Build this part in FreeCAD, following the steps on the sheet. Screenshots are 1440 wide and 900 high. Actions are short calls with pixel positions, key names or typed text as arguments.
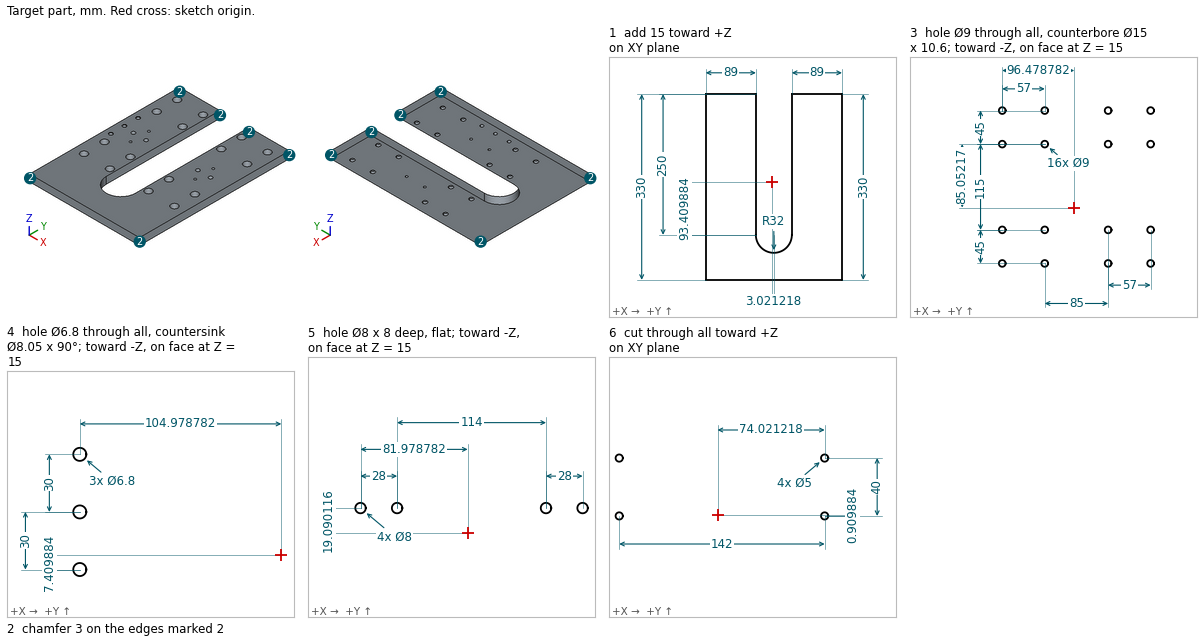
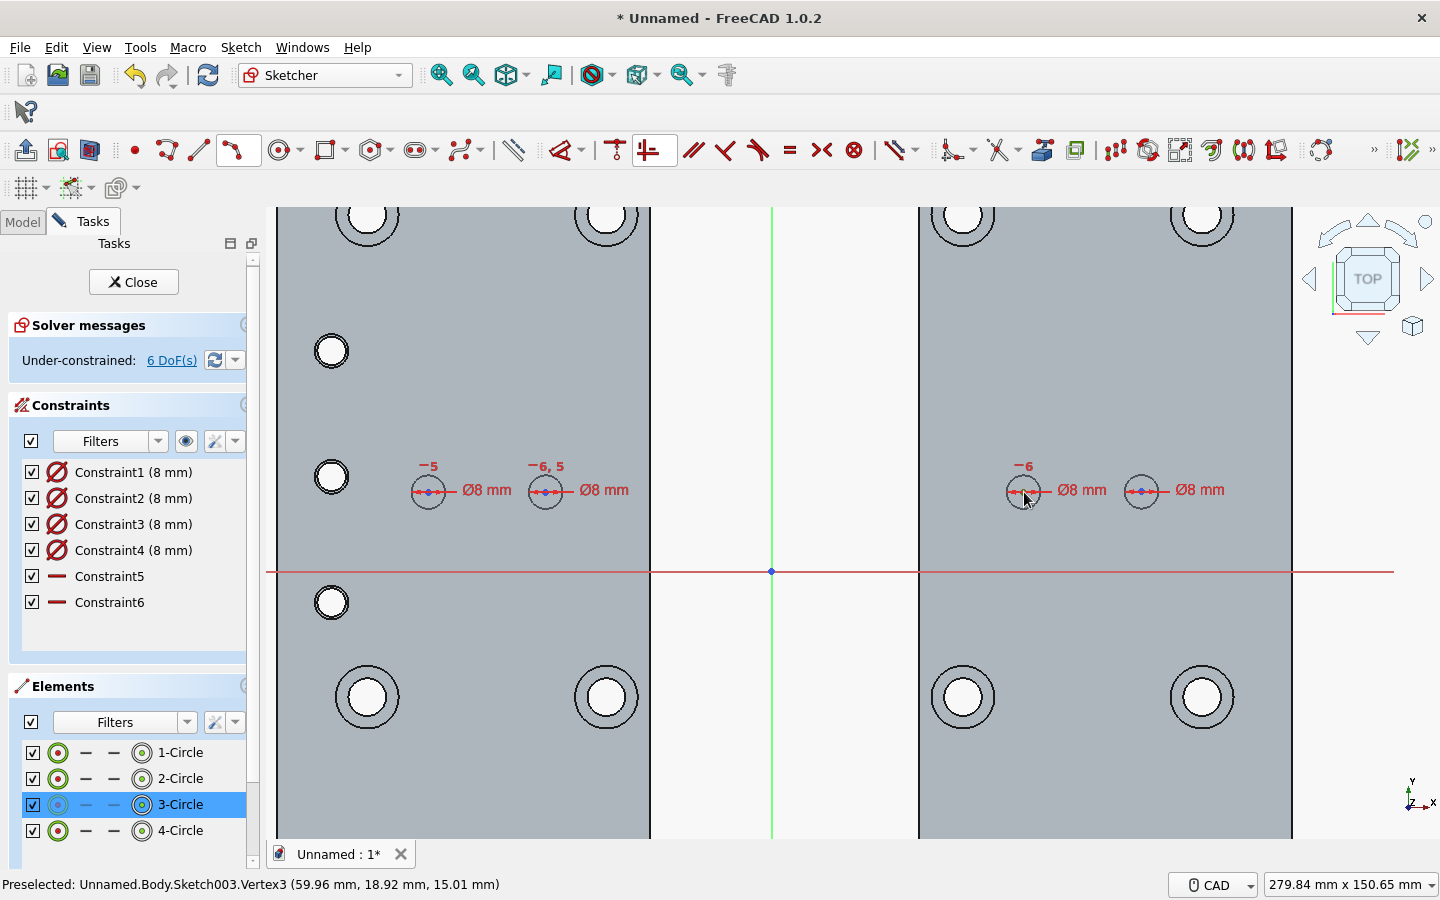
click(1142, 492)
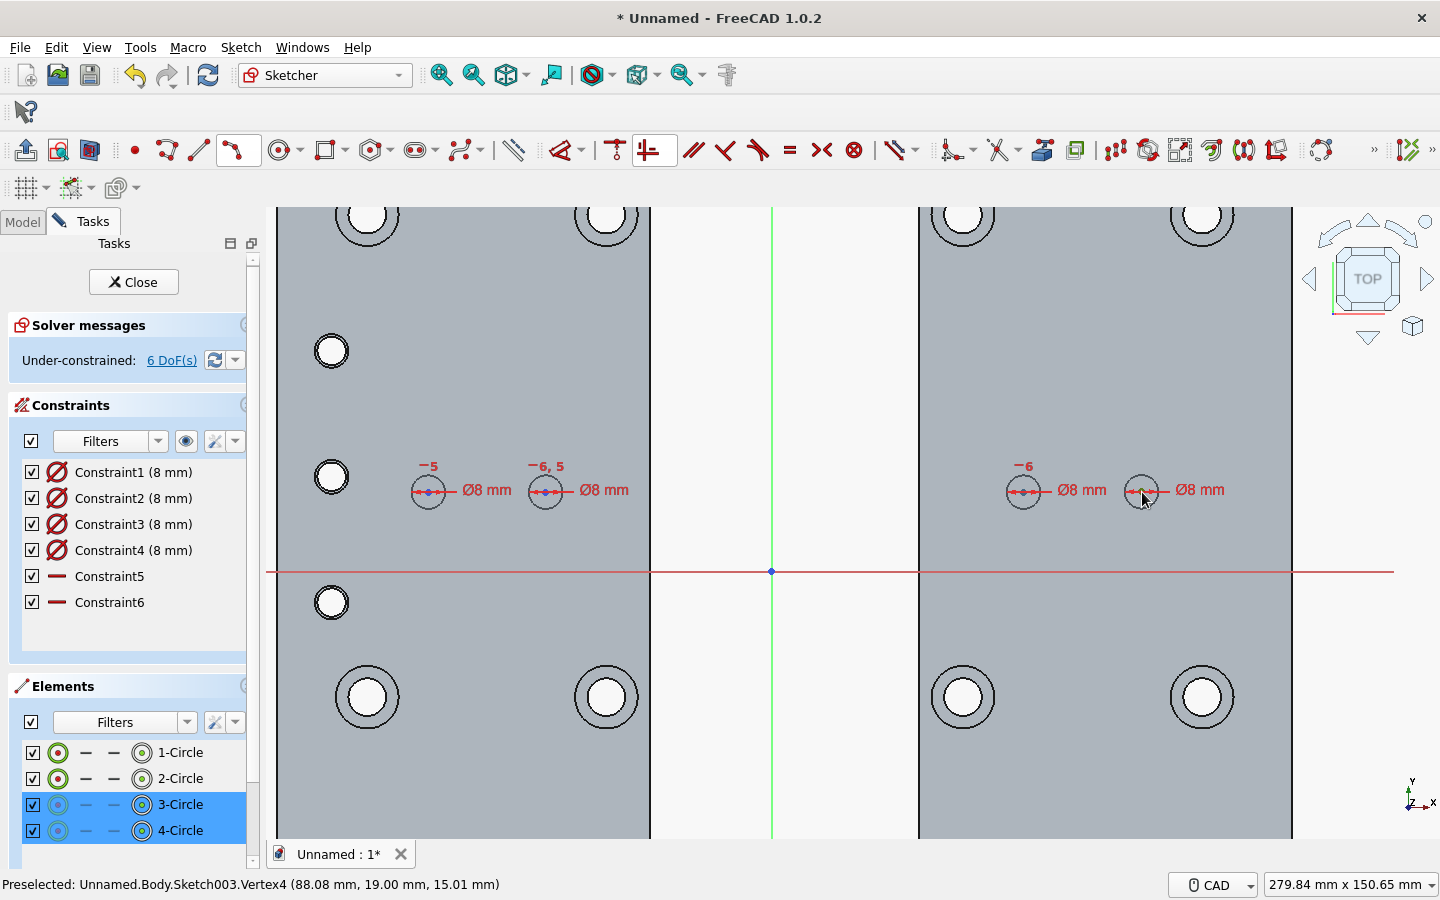
click(672, 150)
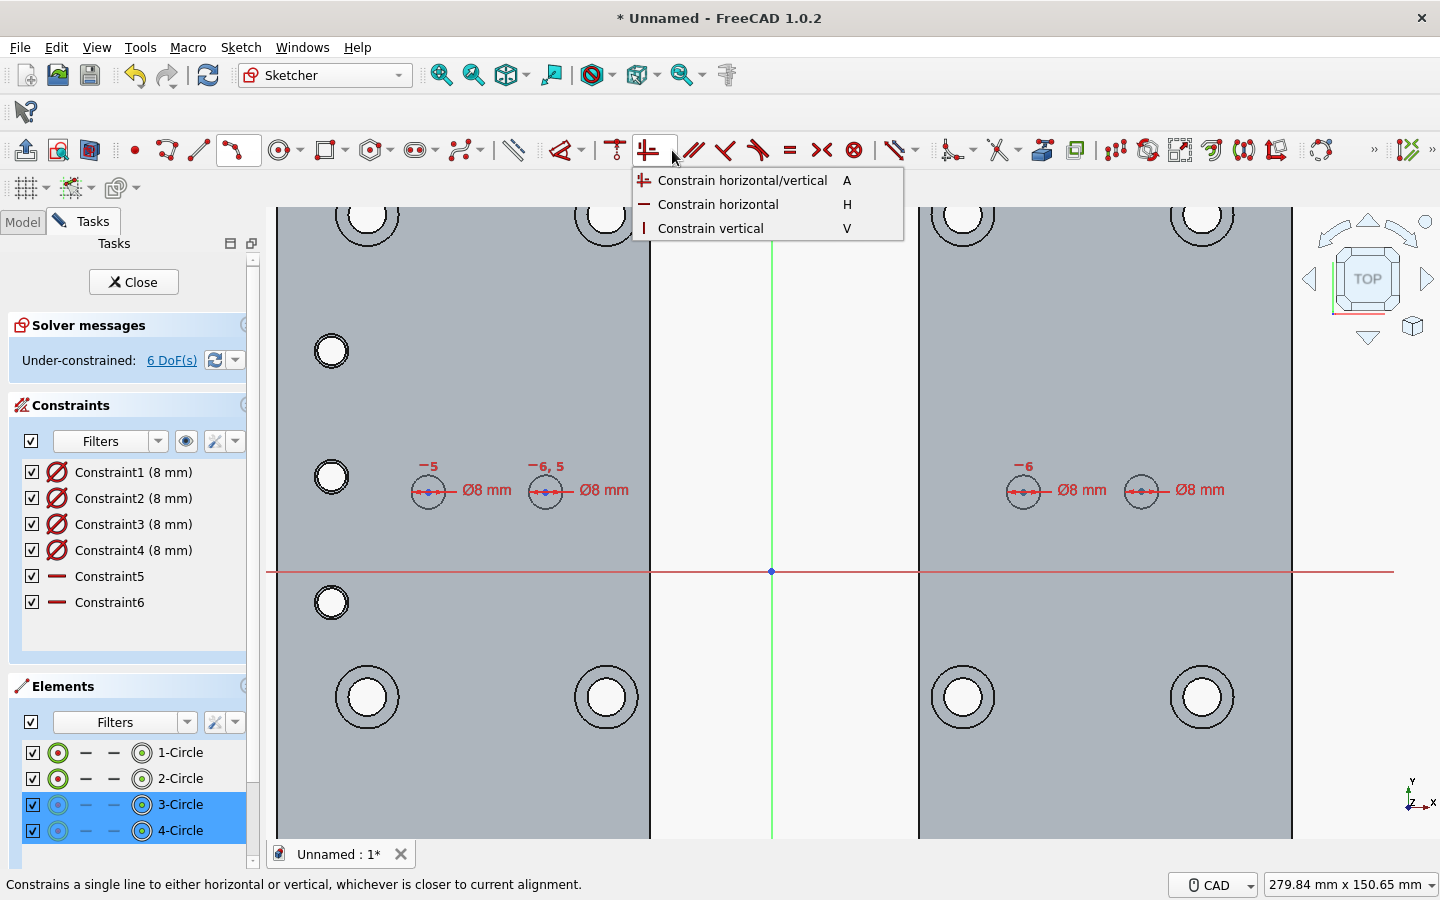
click(768, 204)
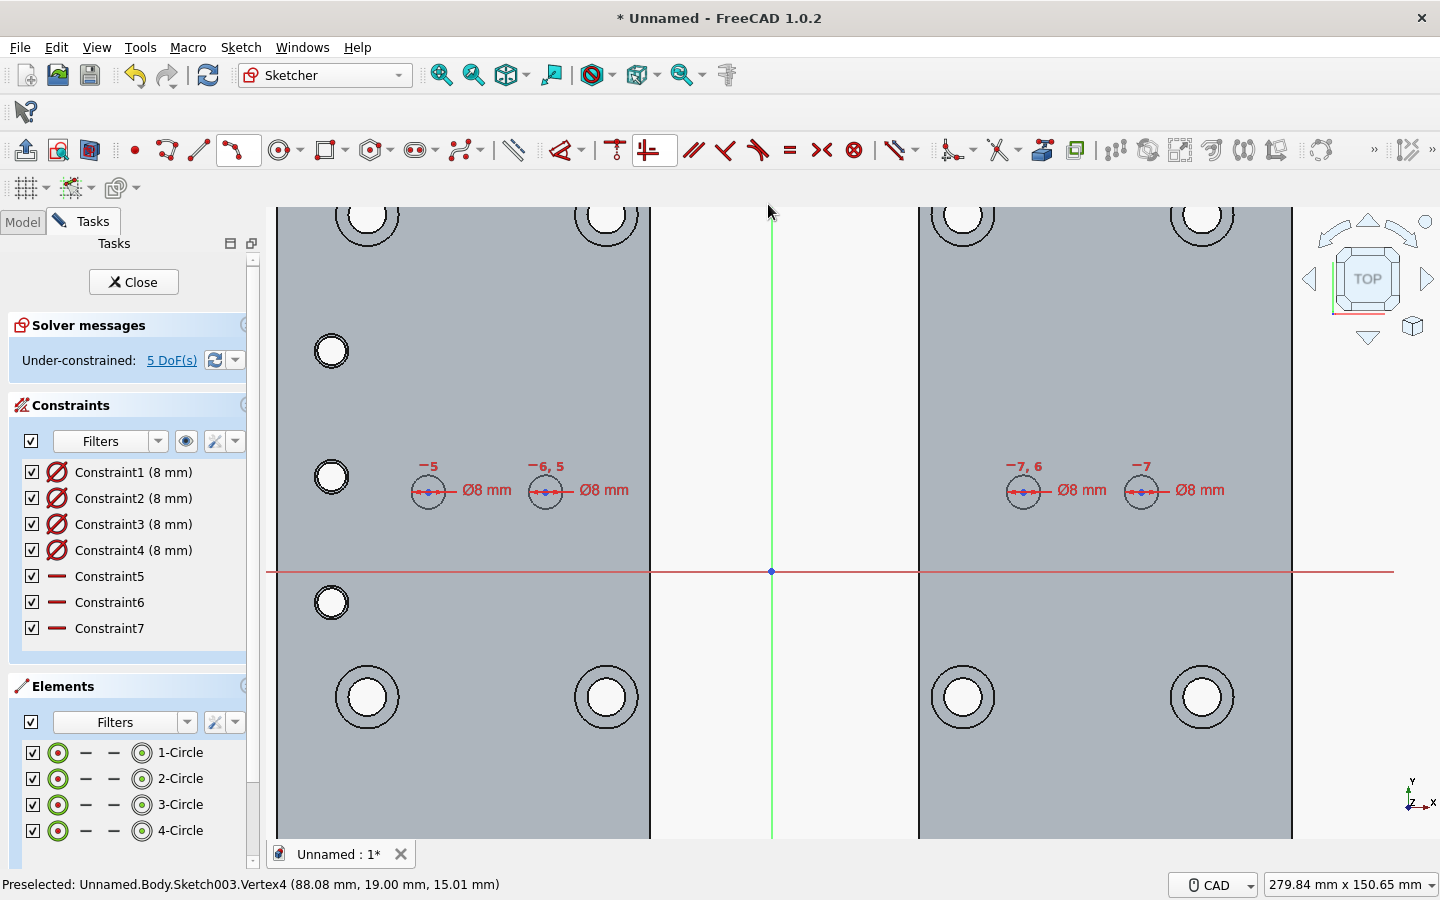
click(560, 150)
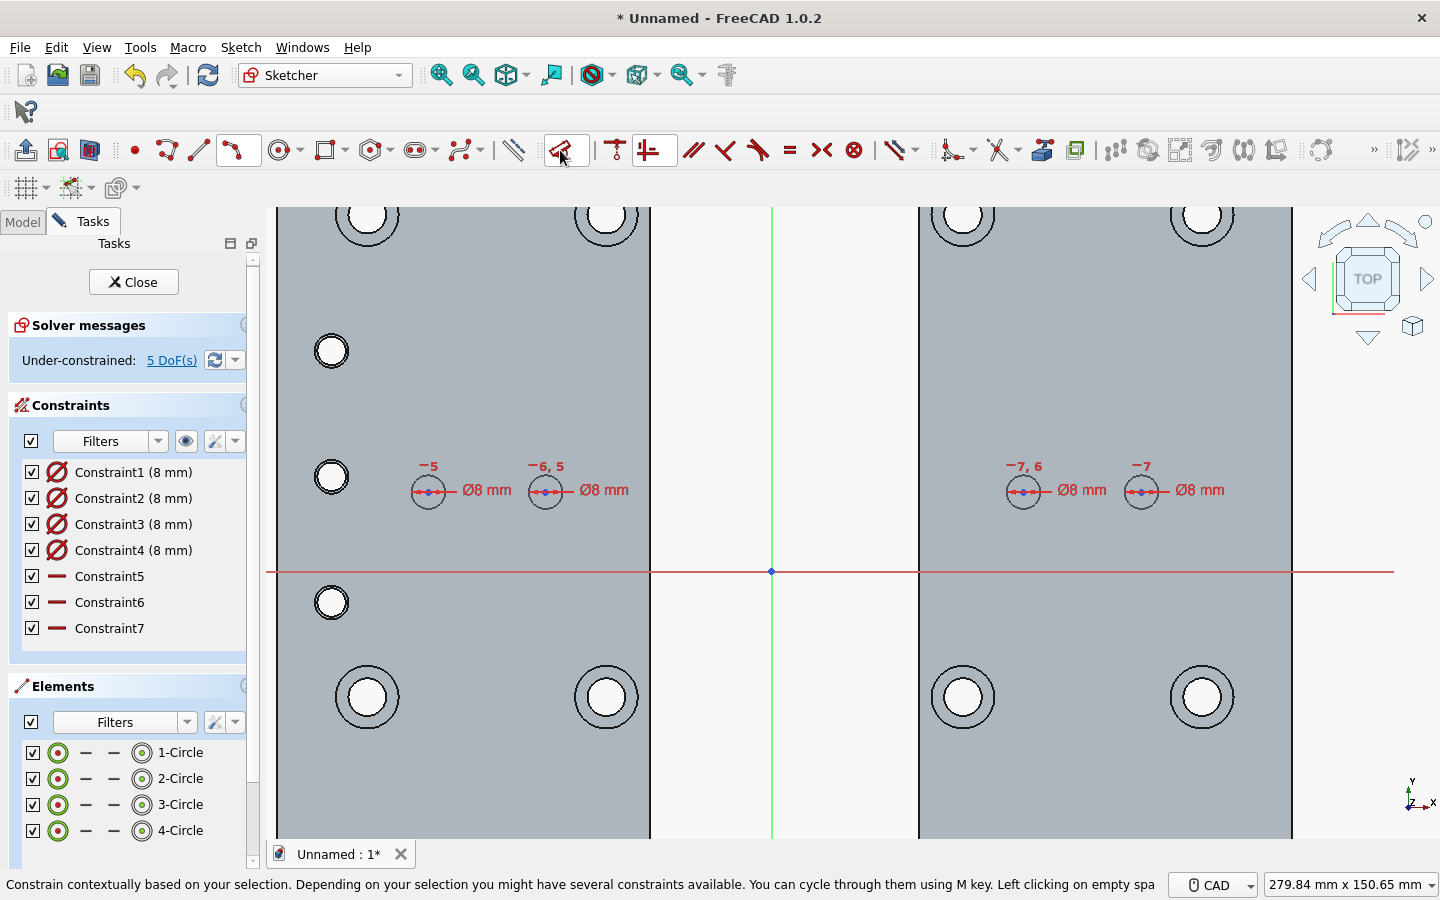
click(428, 492)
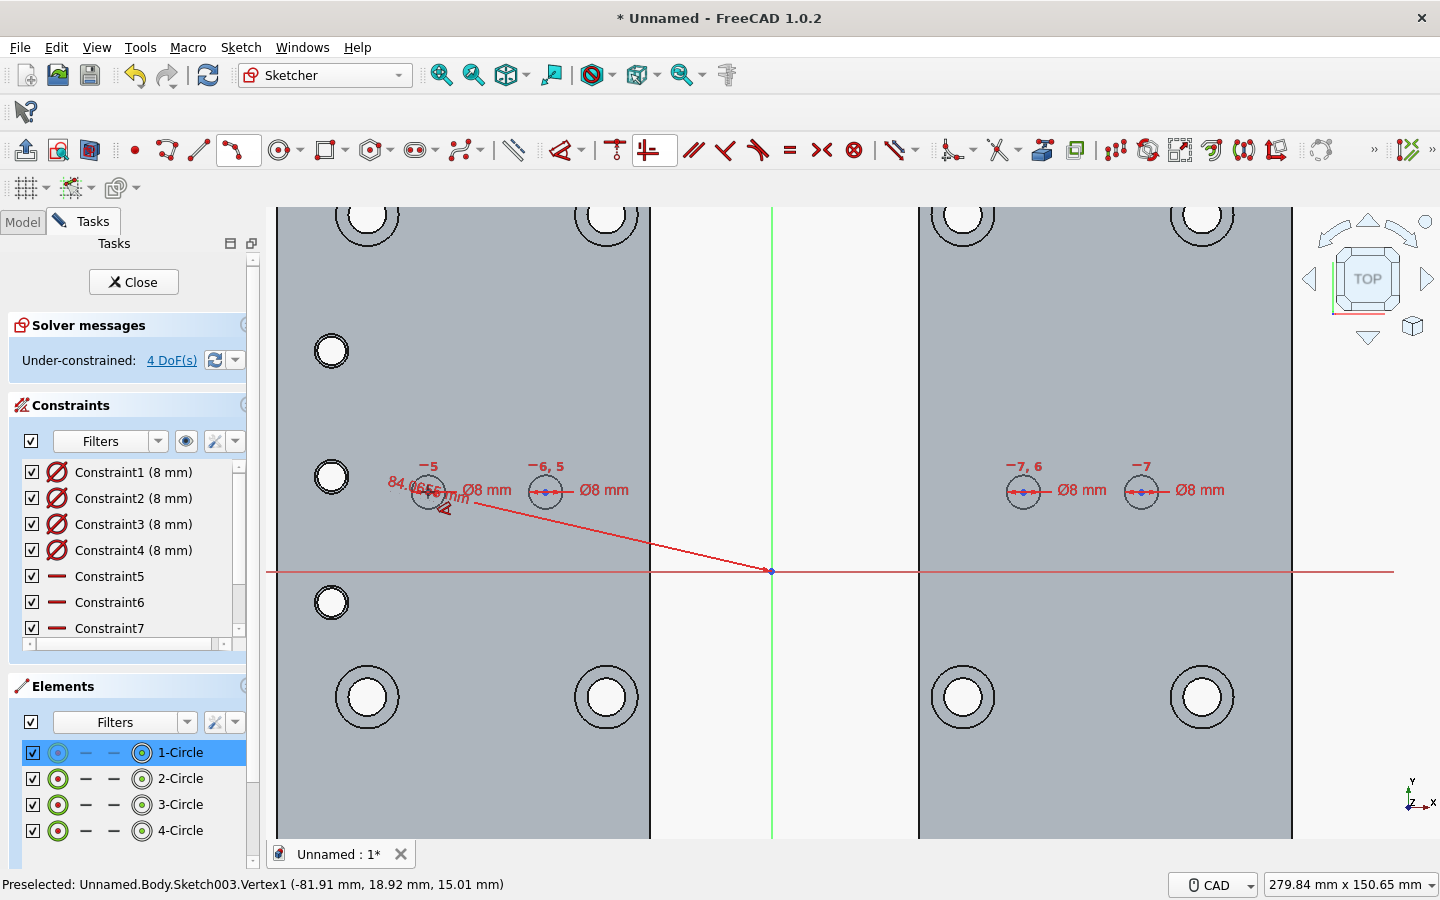
click(546, 492)
click(487, 458)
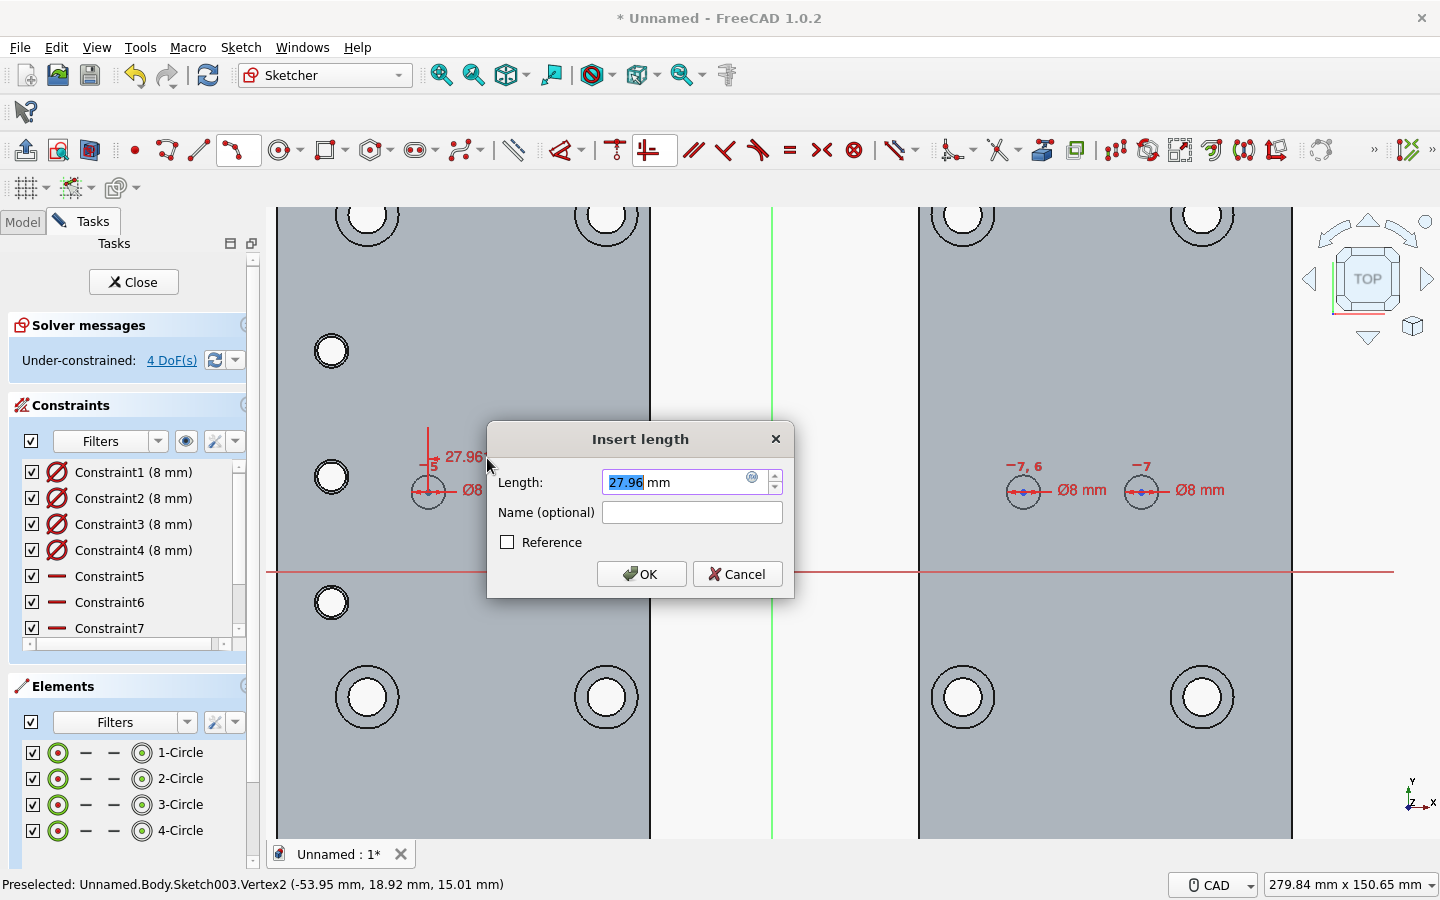
text(28)
key(Return)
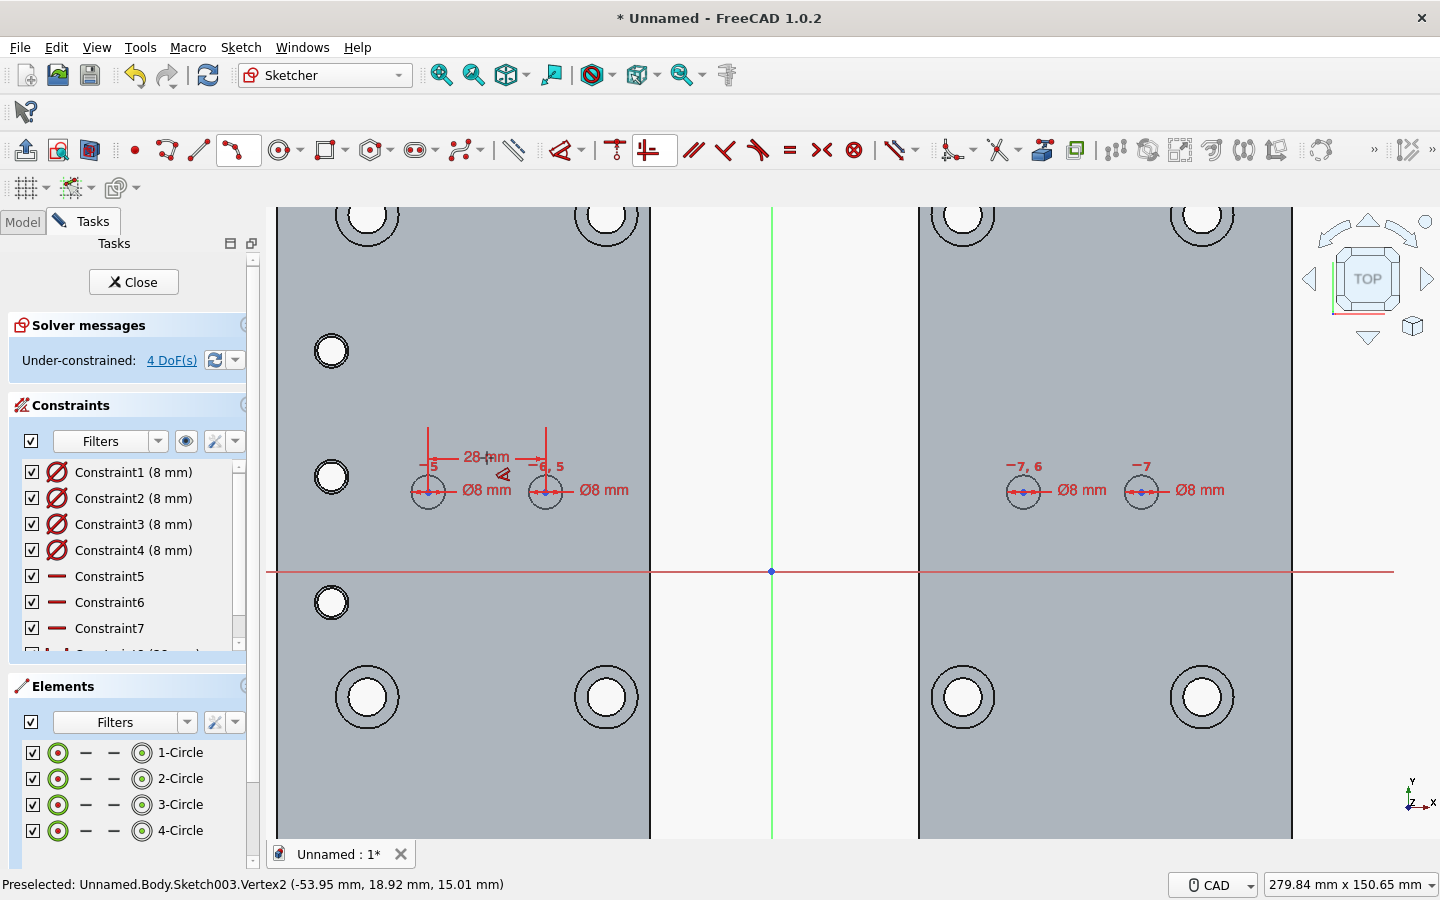
click(1024, 492)